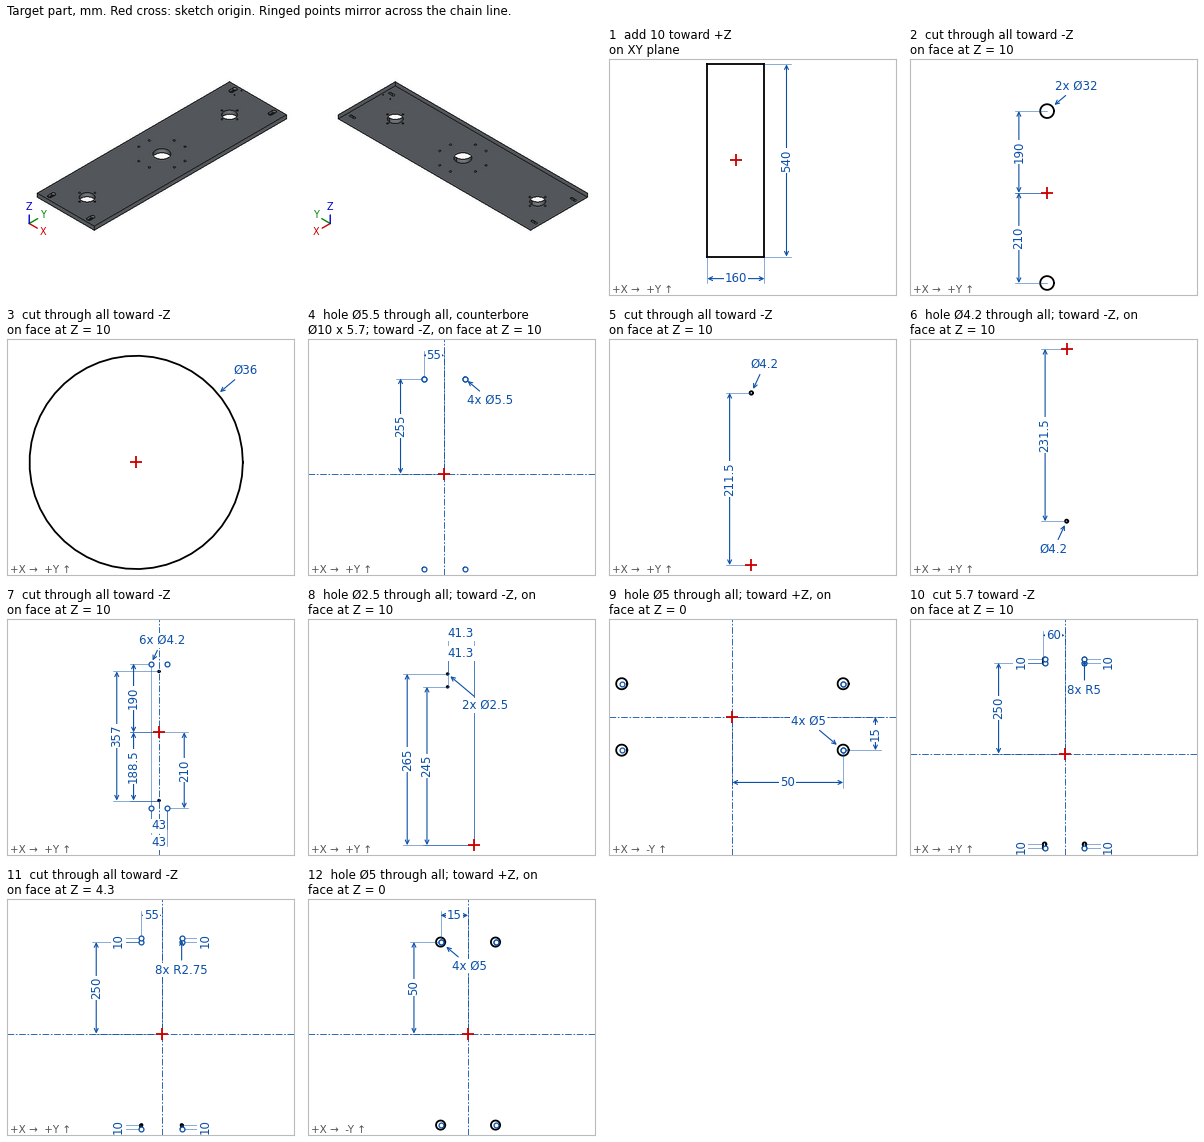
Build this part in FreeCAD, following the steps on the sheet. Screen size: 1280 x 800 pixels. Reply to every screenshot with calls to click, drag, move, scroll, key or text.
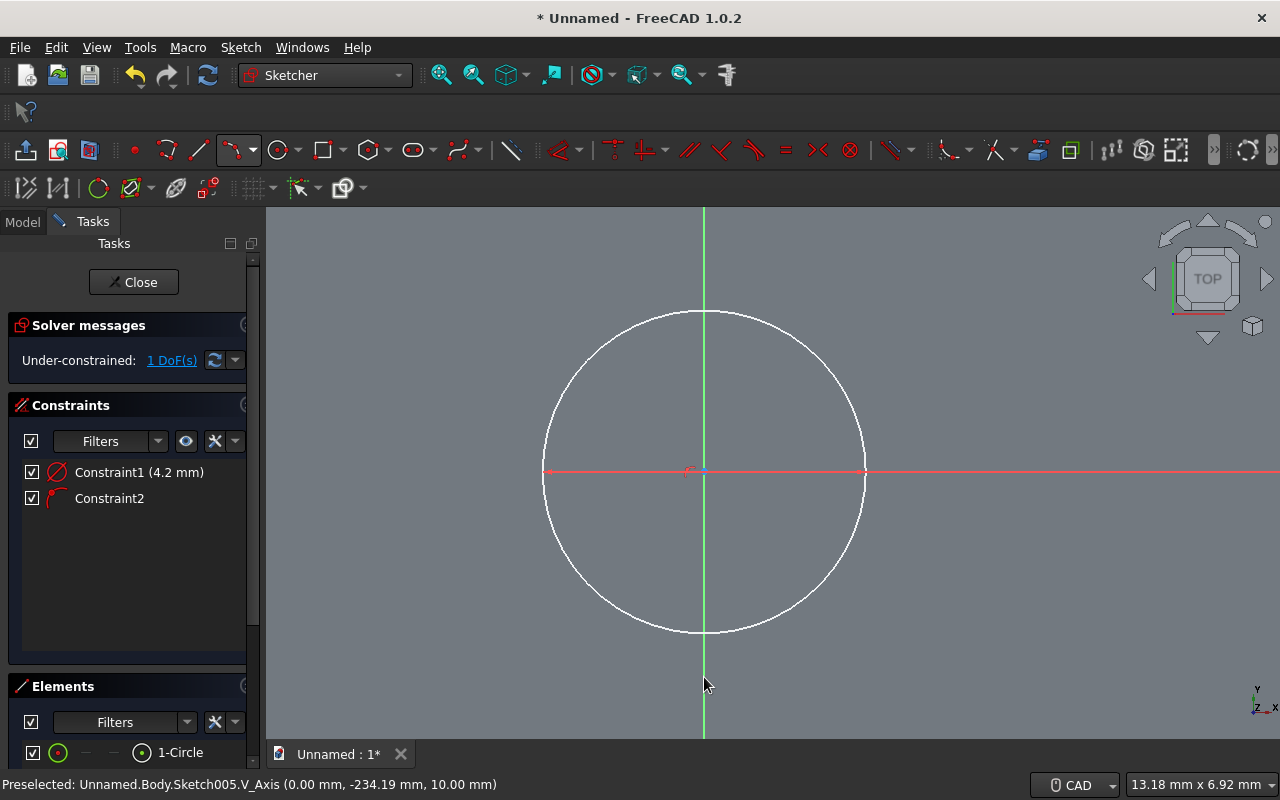
click(558, 150)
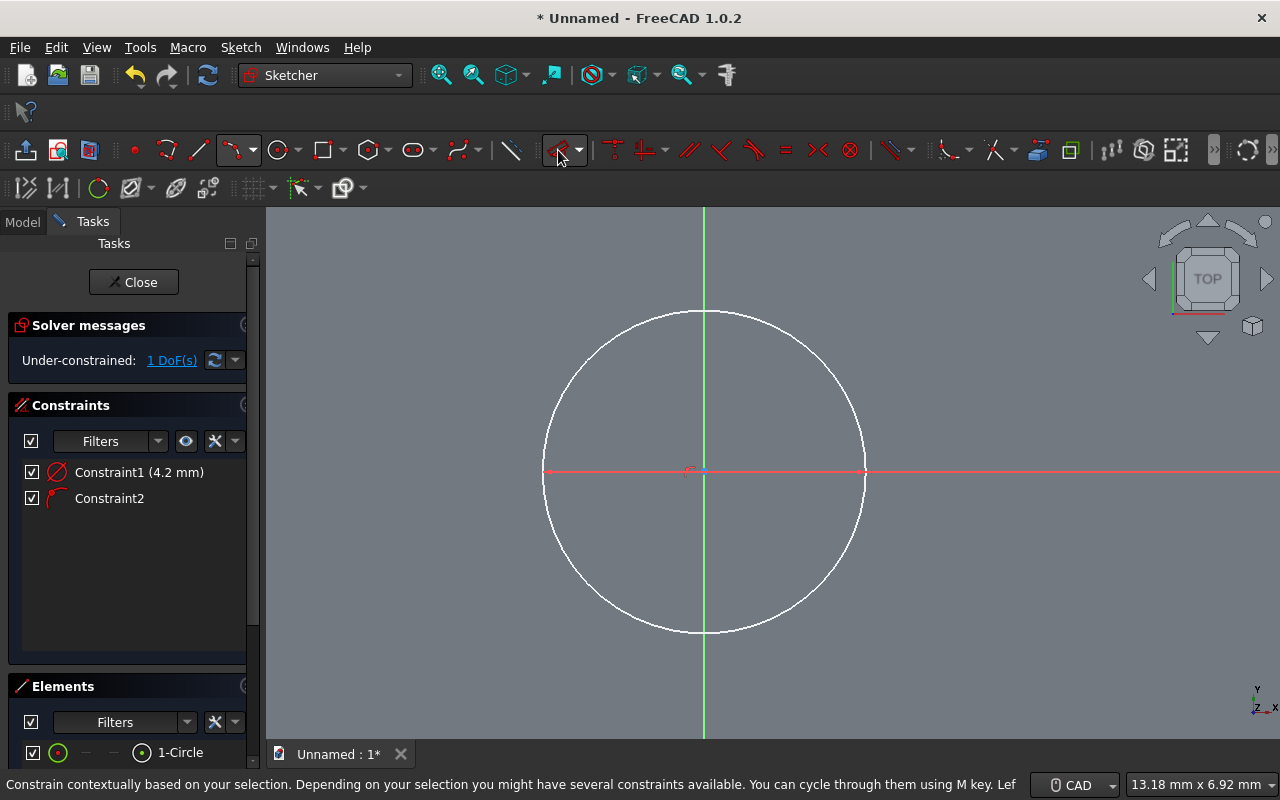
click(704, 472)
click(738, 353)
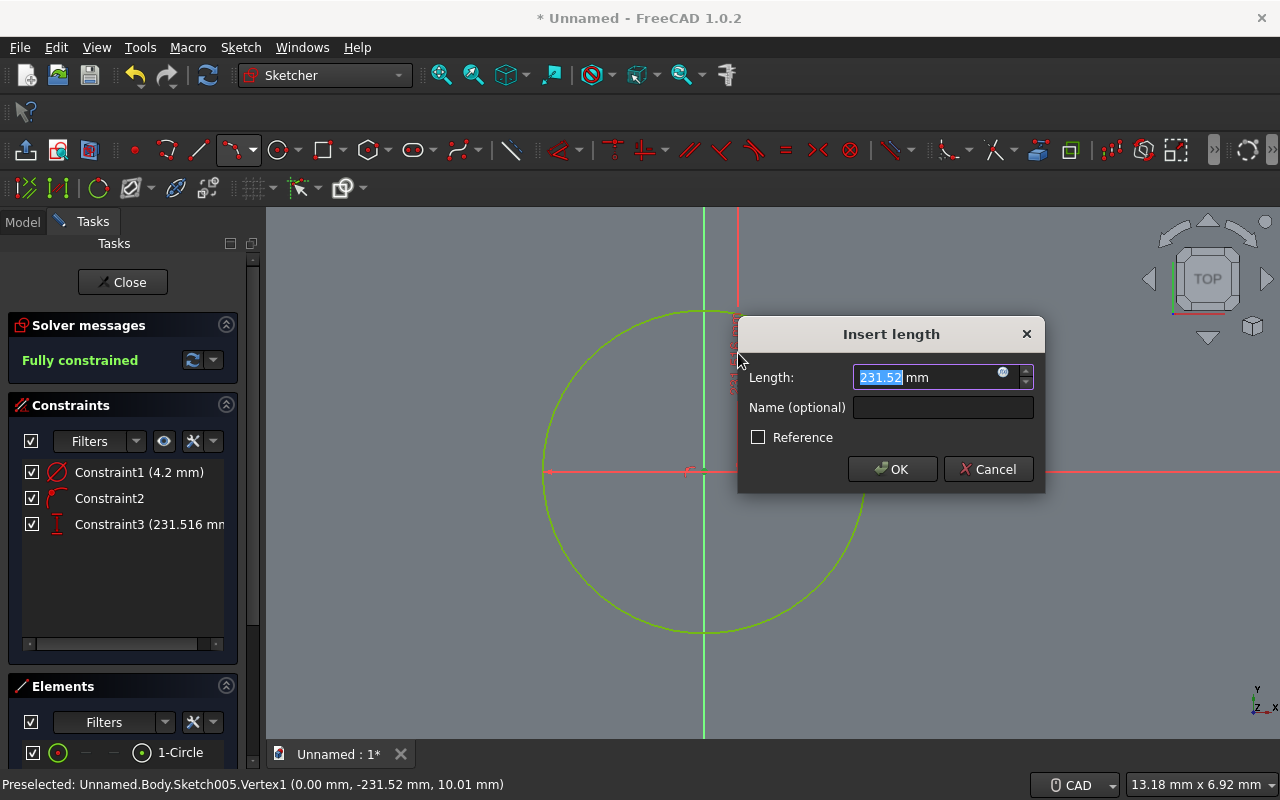
text(231.5)
key(Return)
key(Escape)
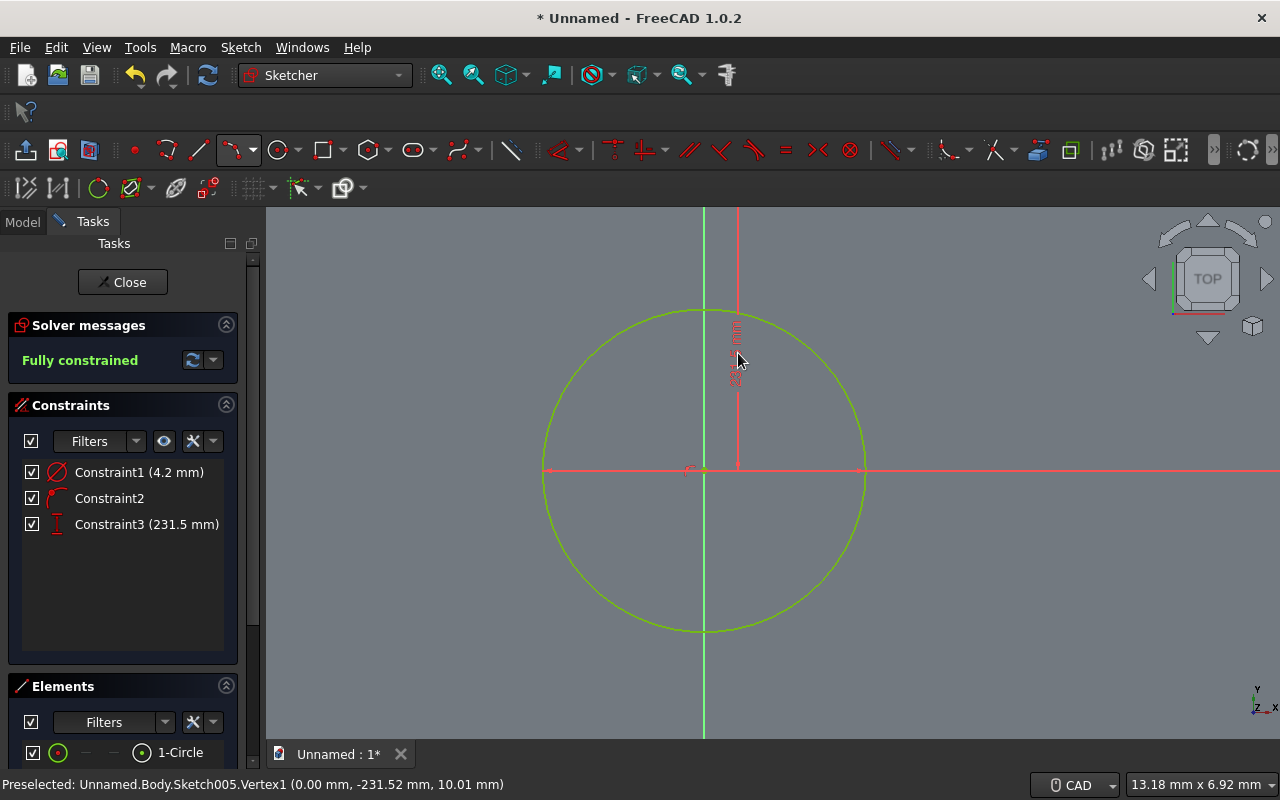
click(123, 282)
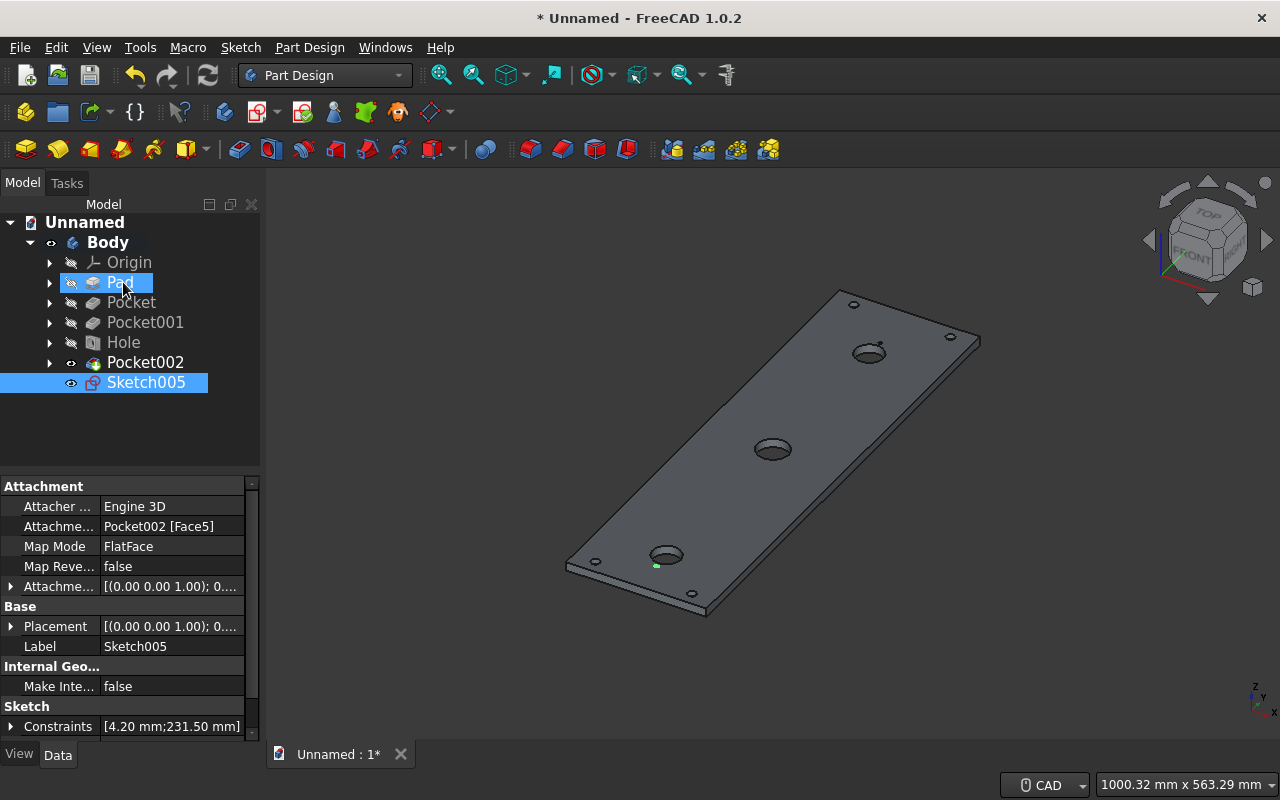
click(272, 150)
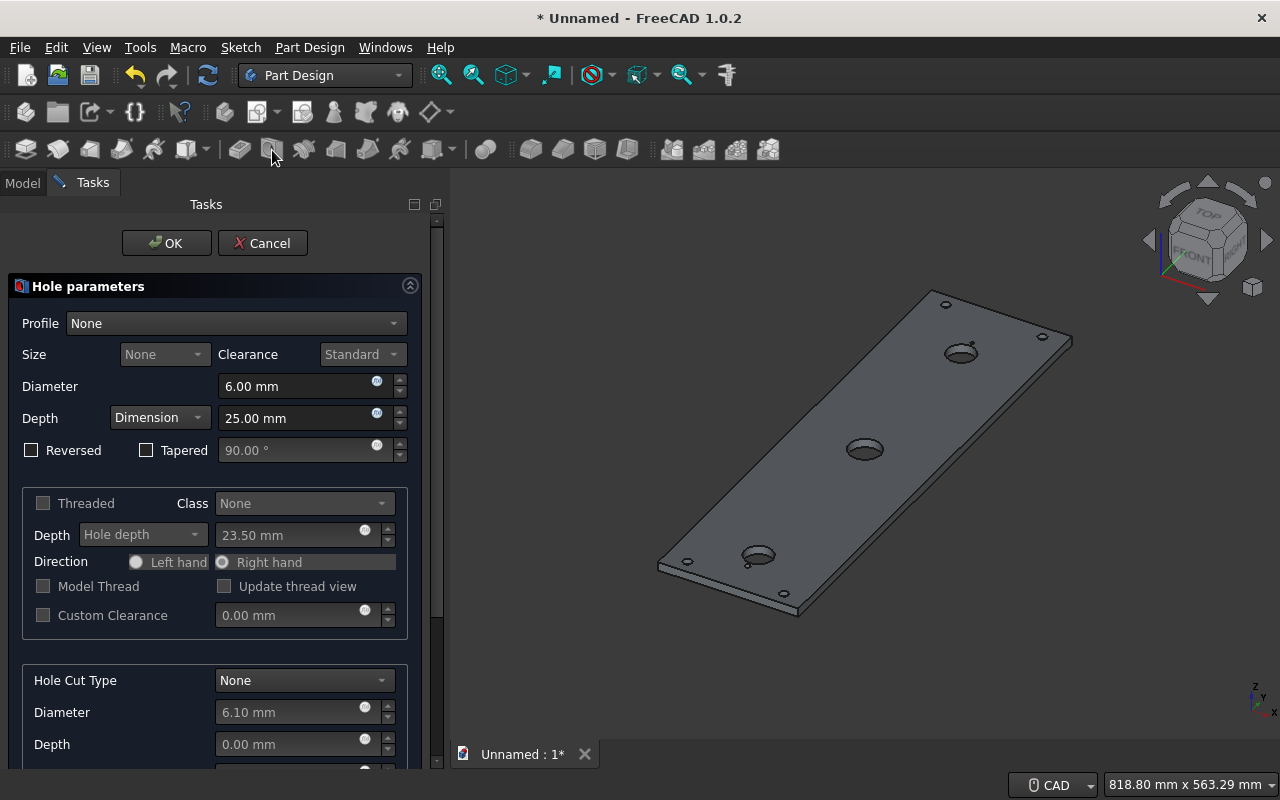
triple_click(305, 386)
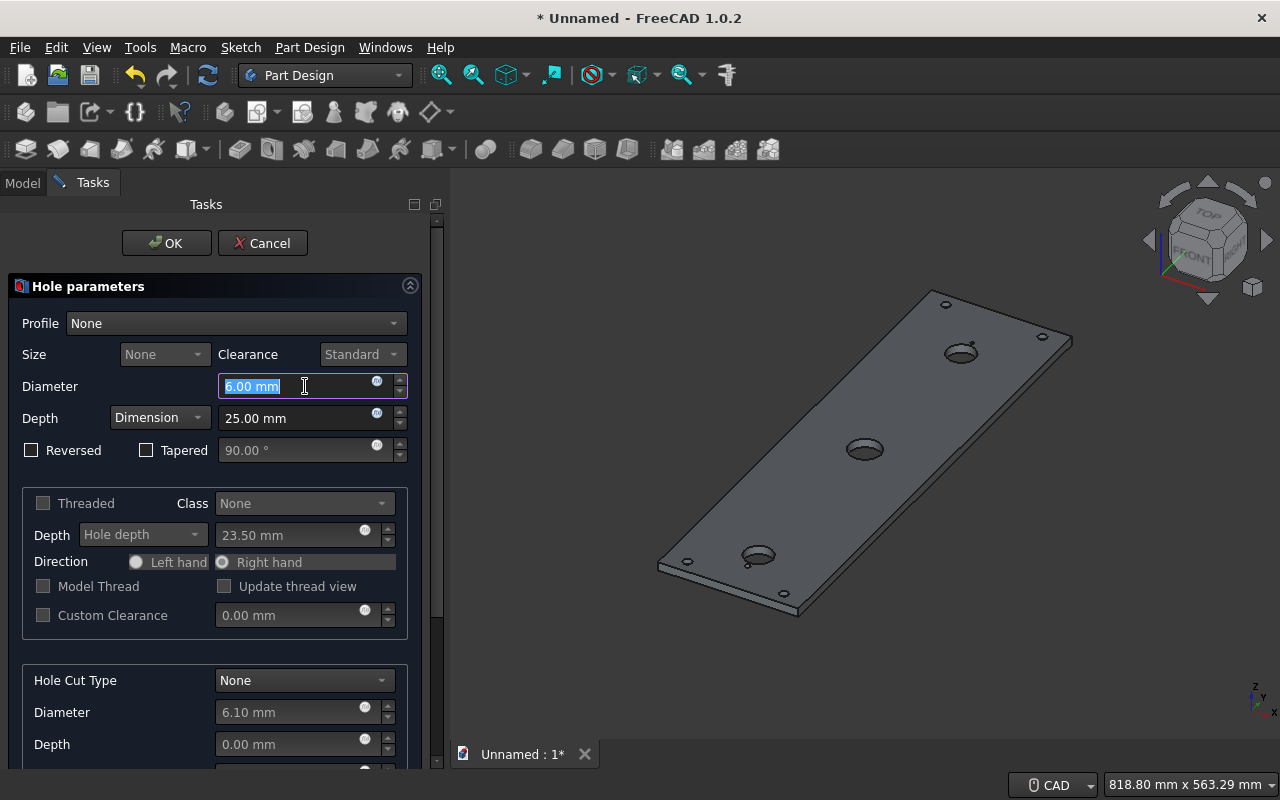
text(4.2)
key(Tab)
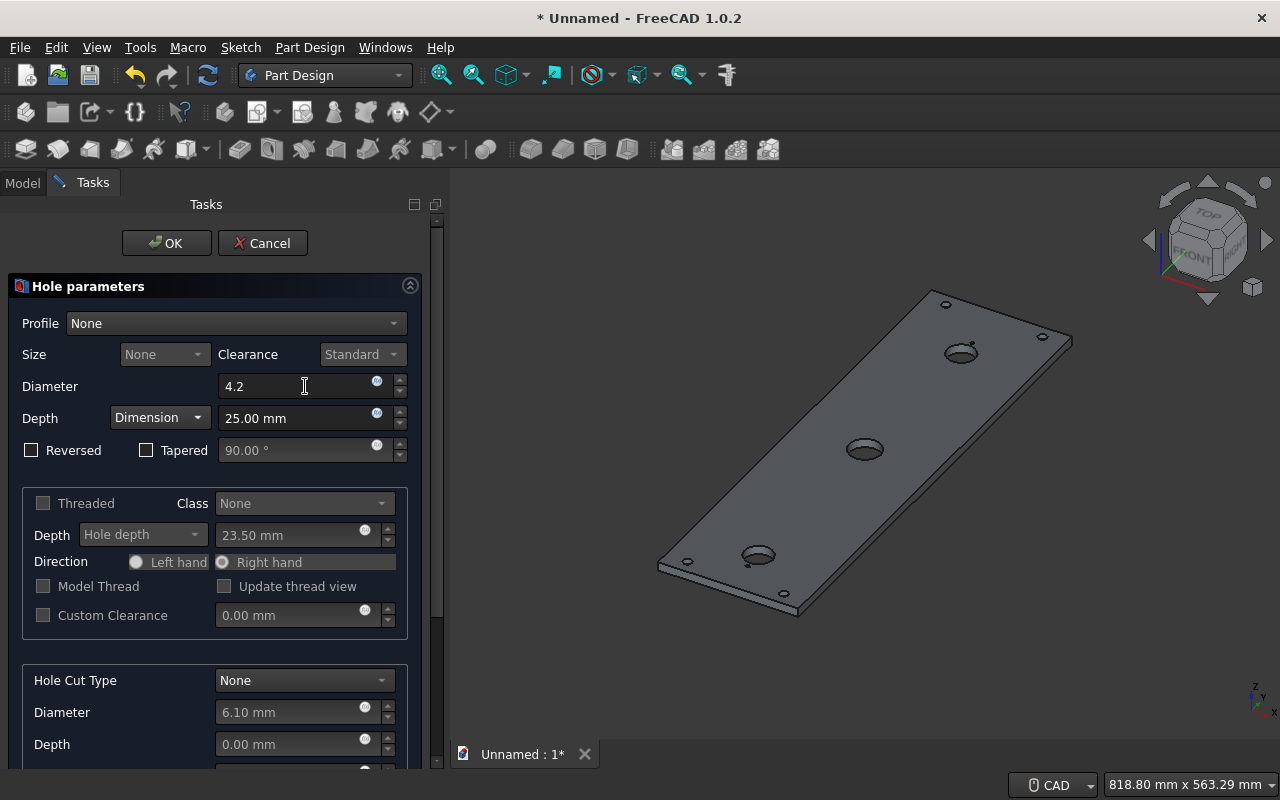
click(161, 418)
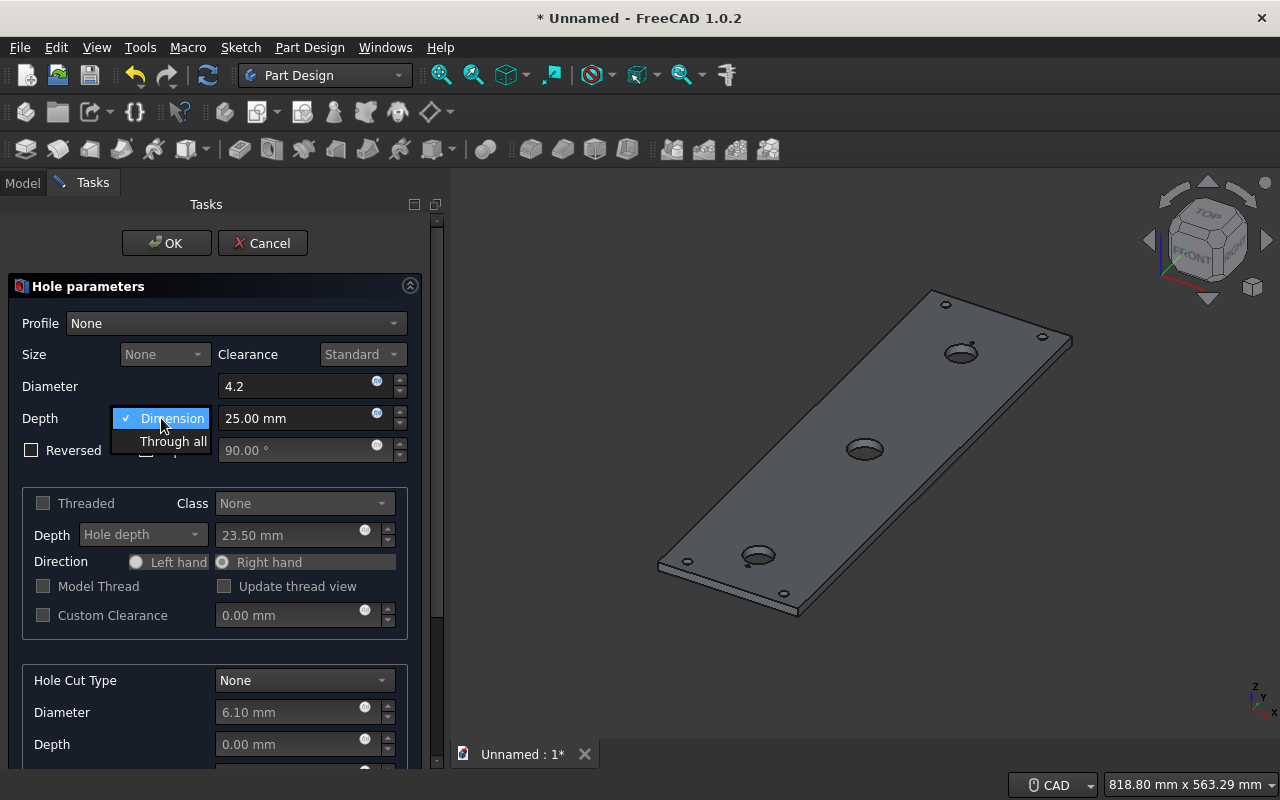
click(160, 442)